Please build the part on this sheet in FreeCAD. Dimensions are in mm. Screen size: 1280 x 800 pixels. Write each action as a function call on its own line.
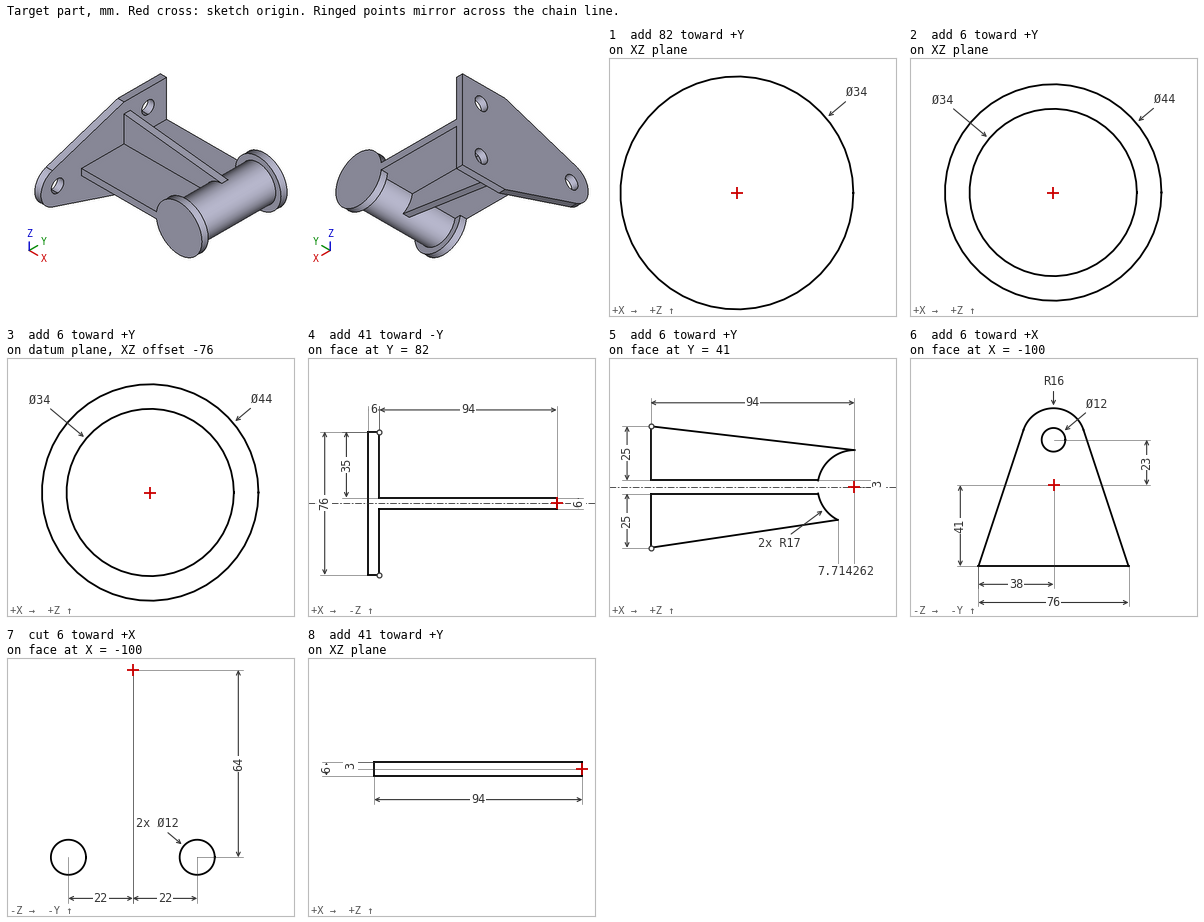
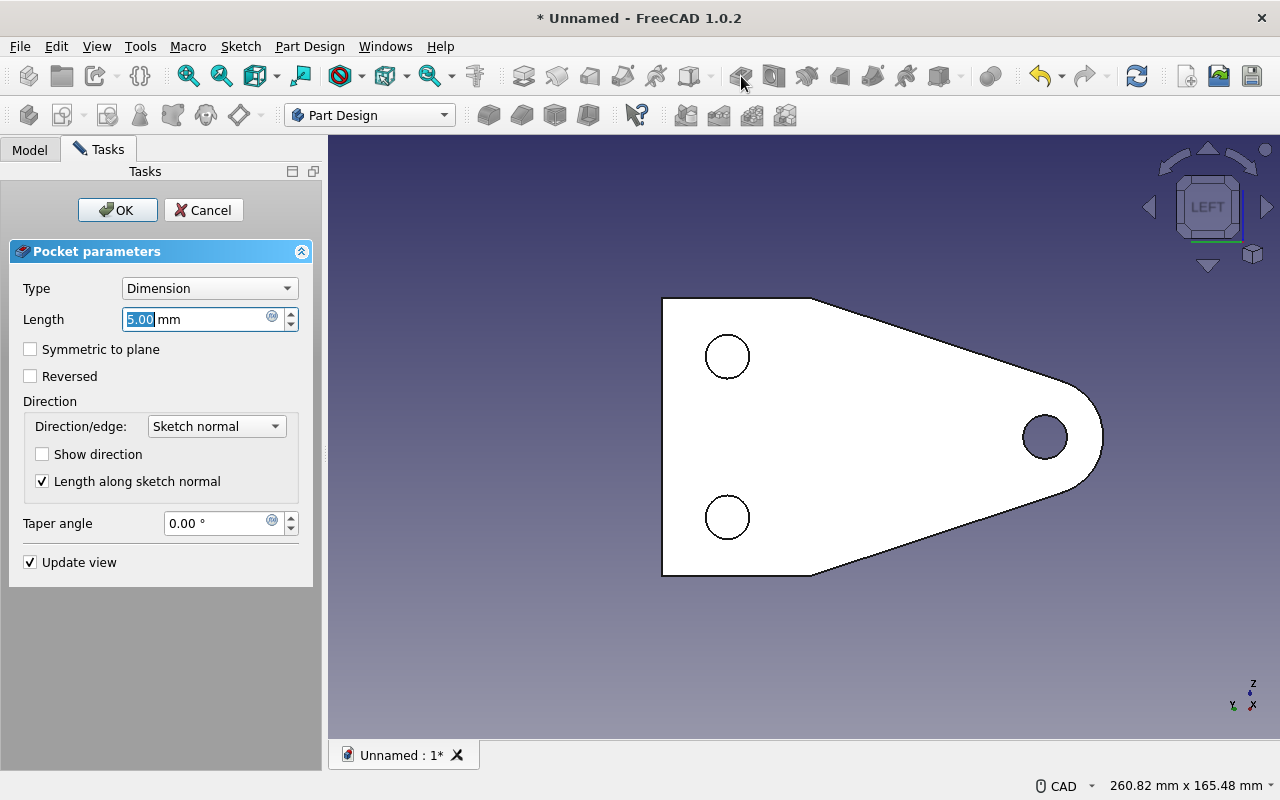
text(6)
key(Tab)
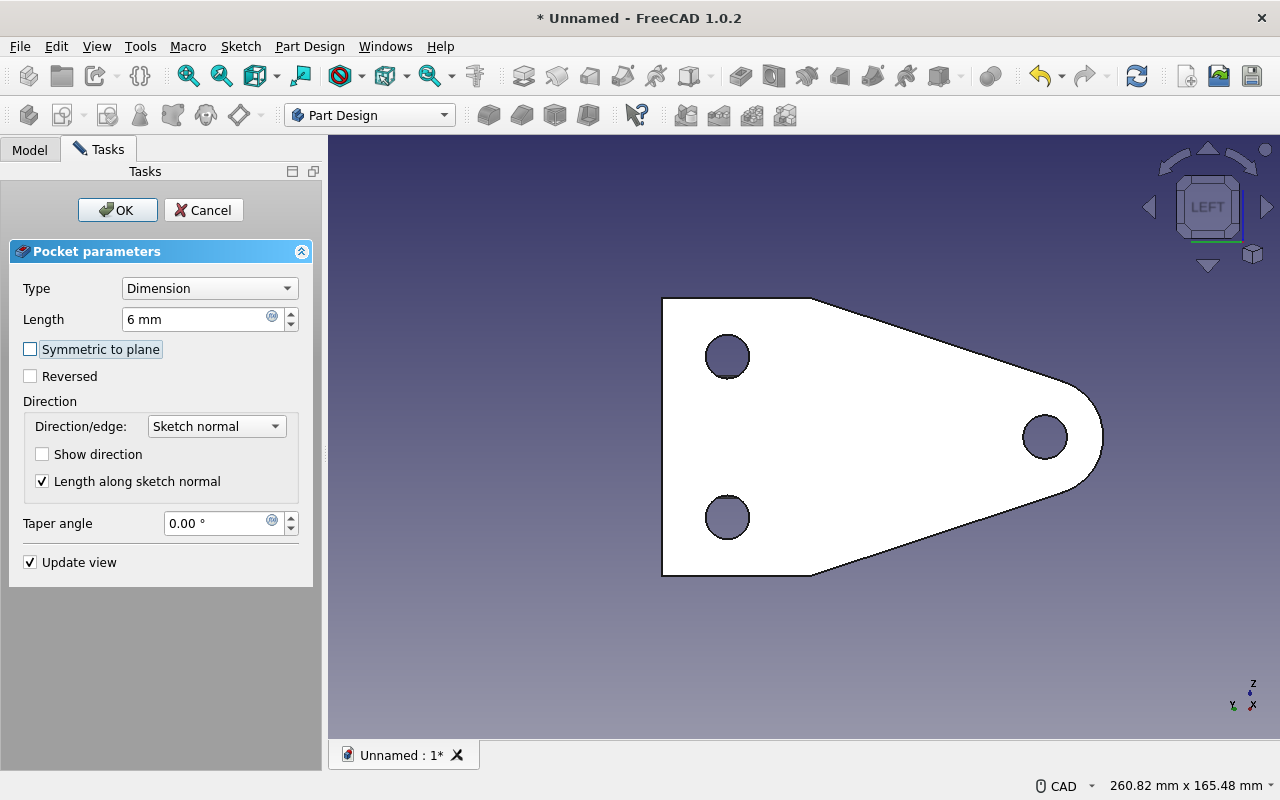
click(118, 210)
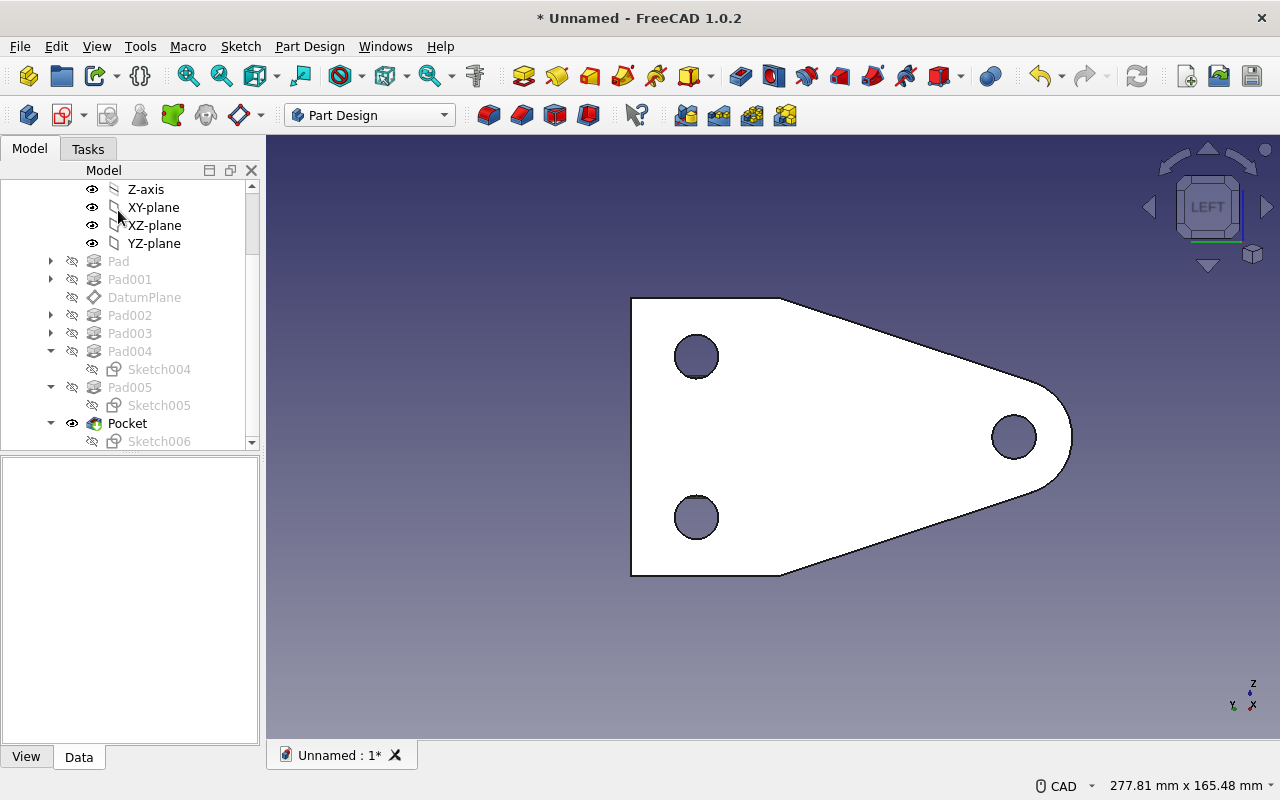
click(62, 116)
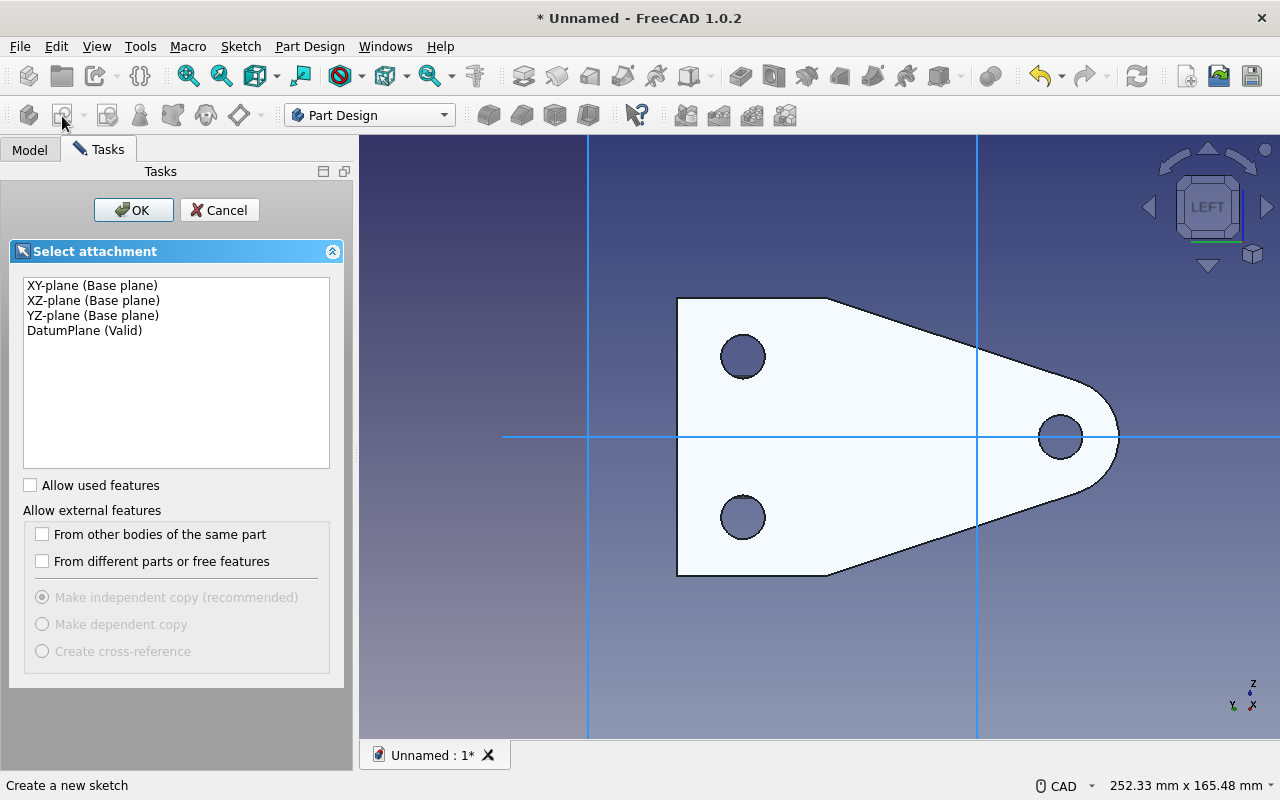
click(84, 300)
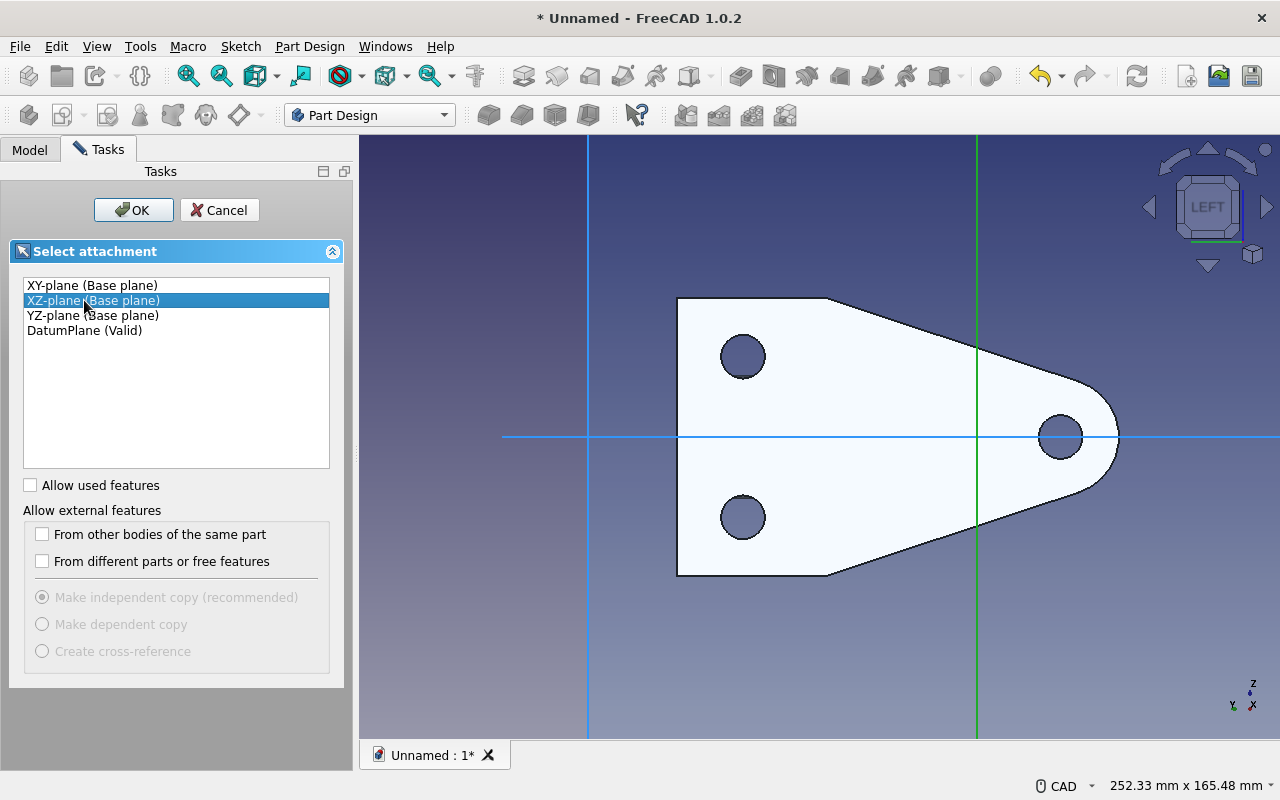
click(134, 210)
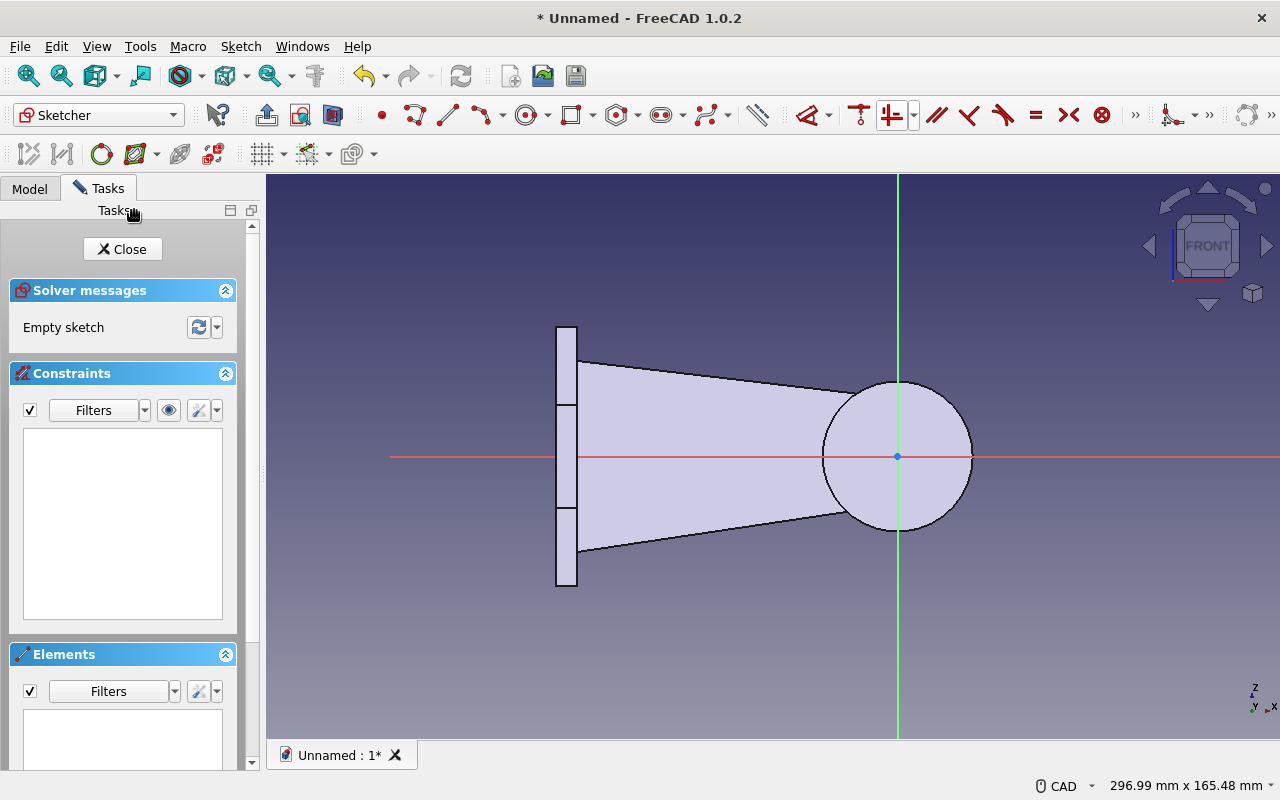
click(333, 116)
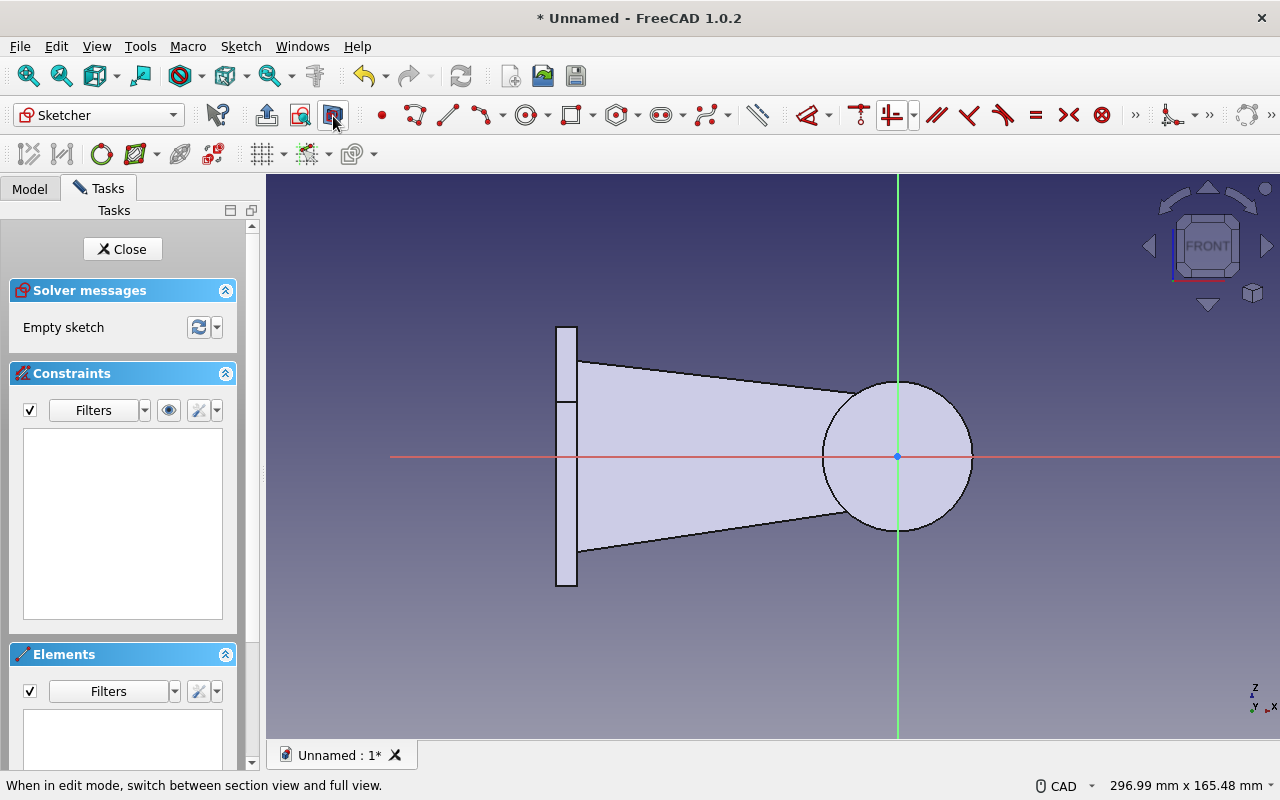
scroll(777, 457, up, 3)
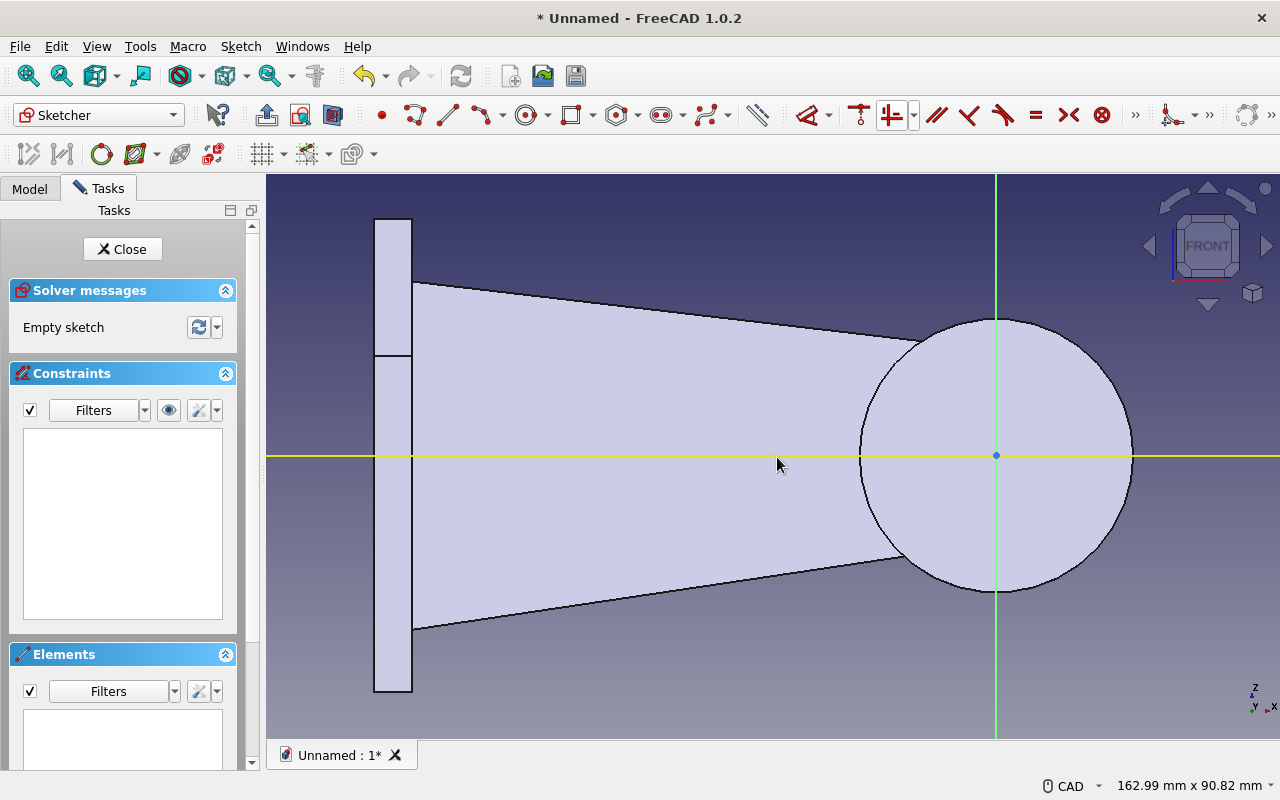
click(570, 116)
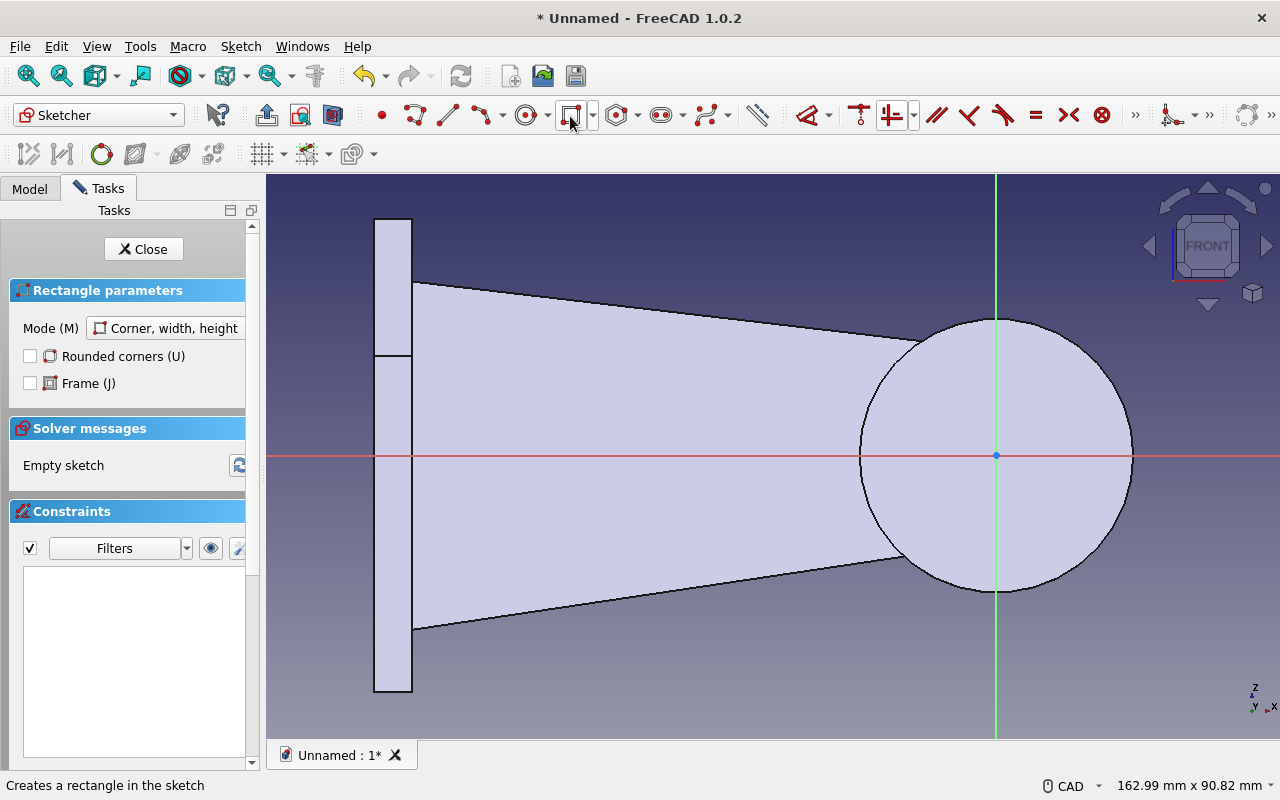
click(412, 437)
click(996, 474)
key(Escape)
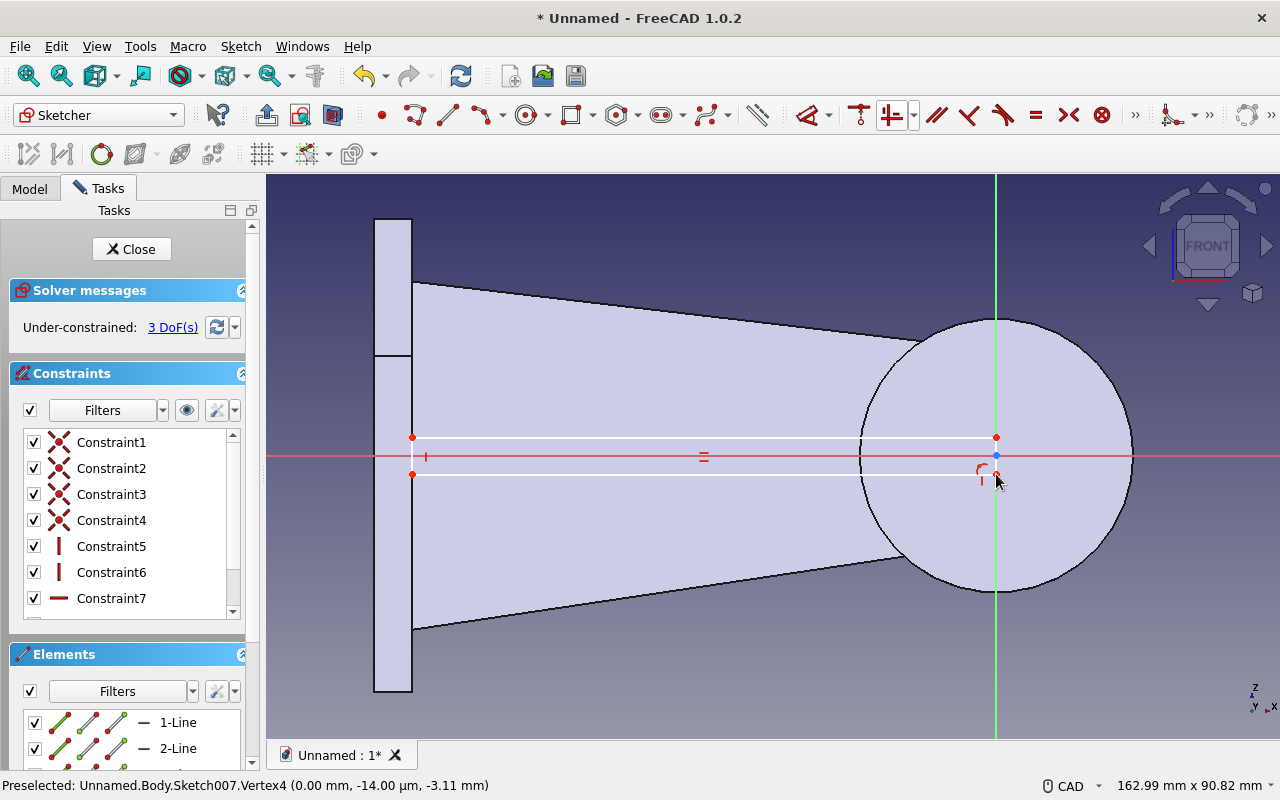
key(d)